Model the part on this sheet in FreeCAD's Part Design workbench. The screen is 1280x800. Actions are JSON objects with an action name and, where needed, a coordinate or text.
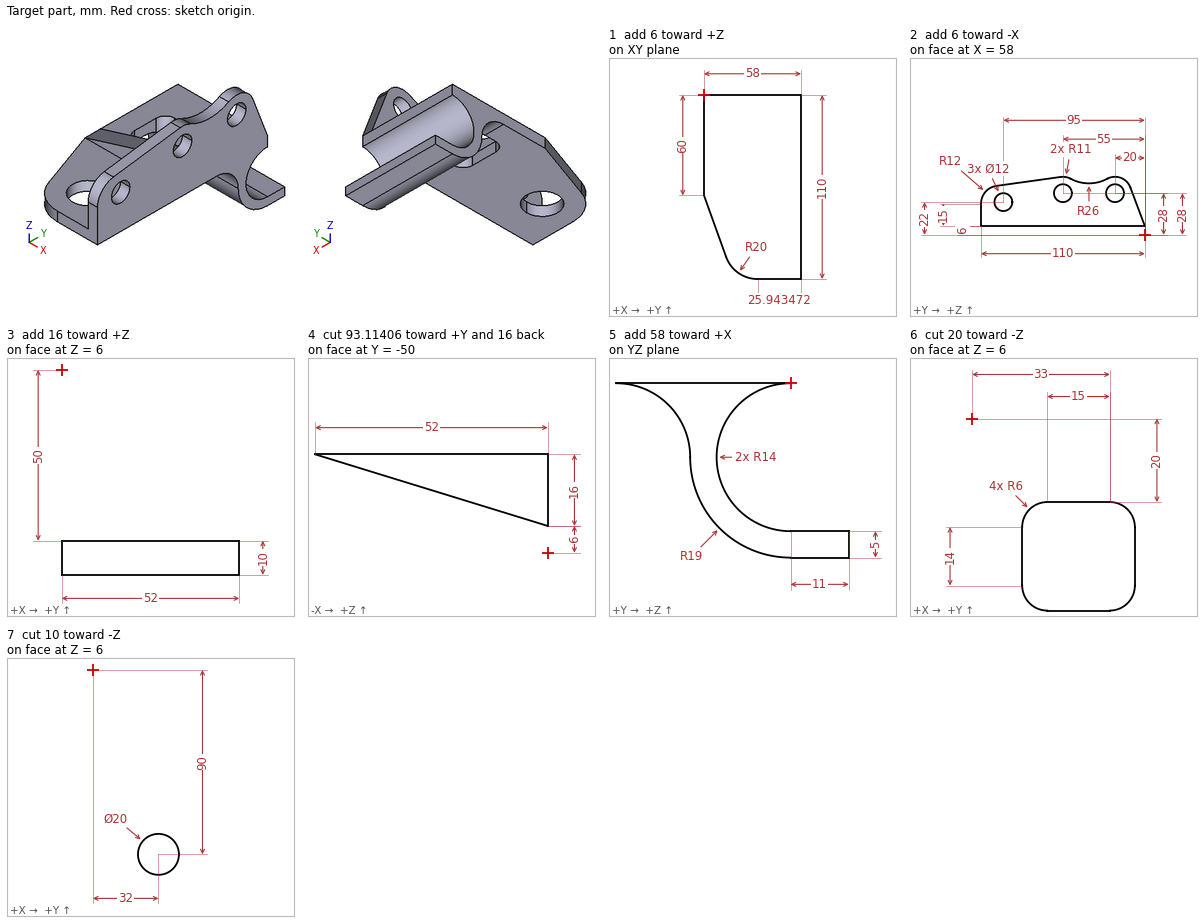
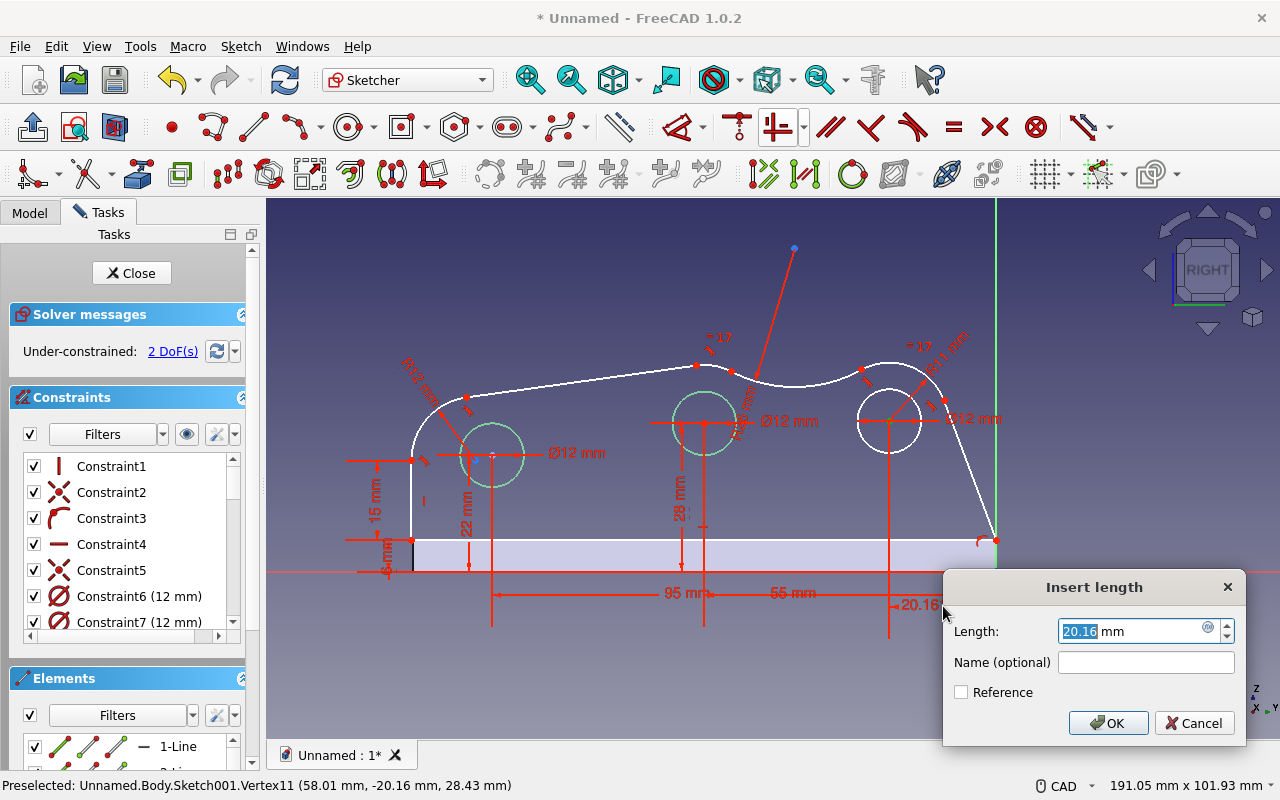
{"action": "type", "text": "20"}
{"action": "key", "text": "Return"}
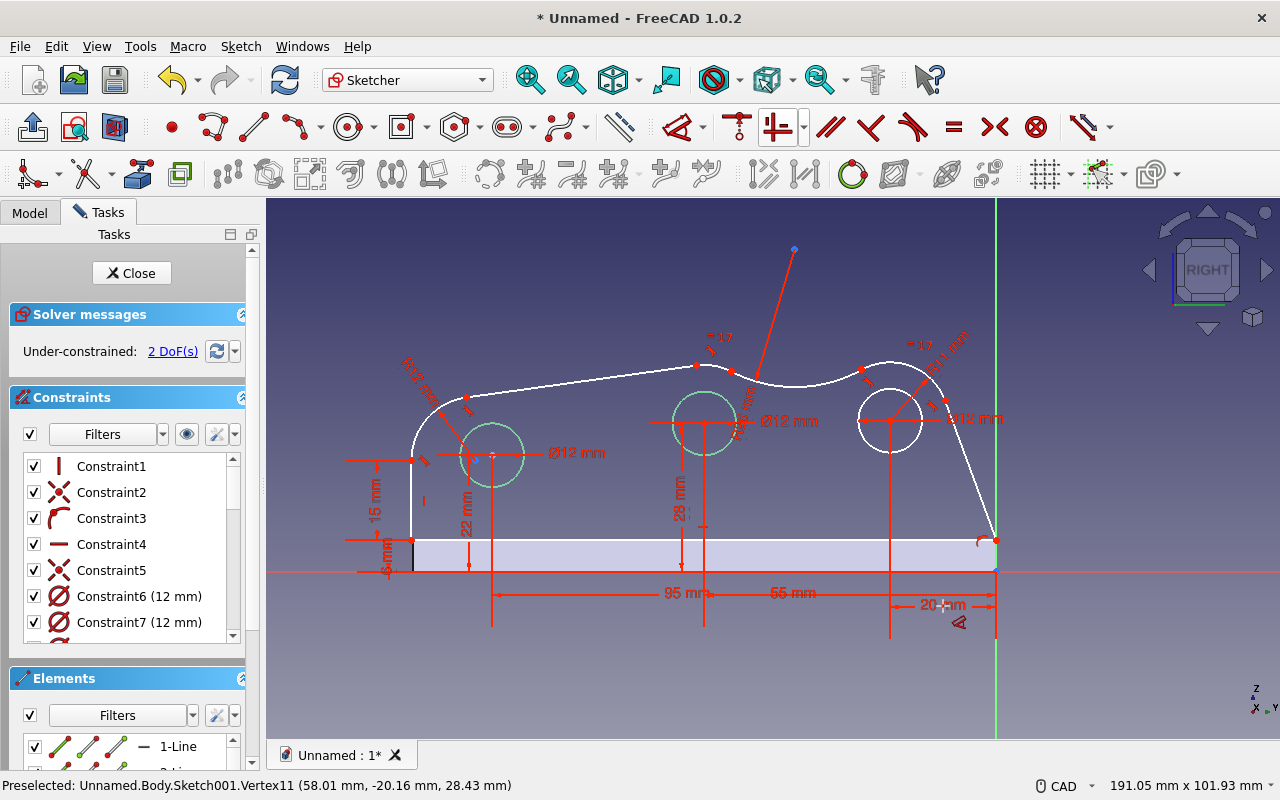
{"action": "left_click", "coordinate": [890, 421]}
{"action": "left_click", "coordinate": [1030, 496]}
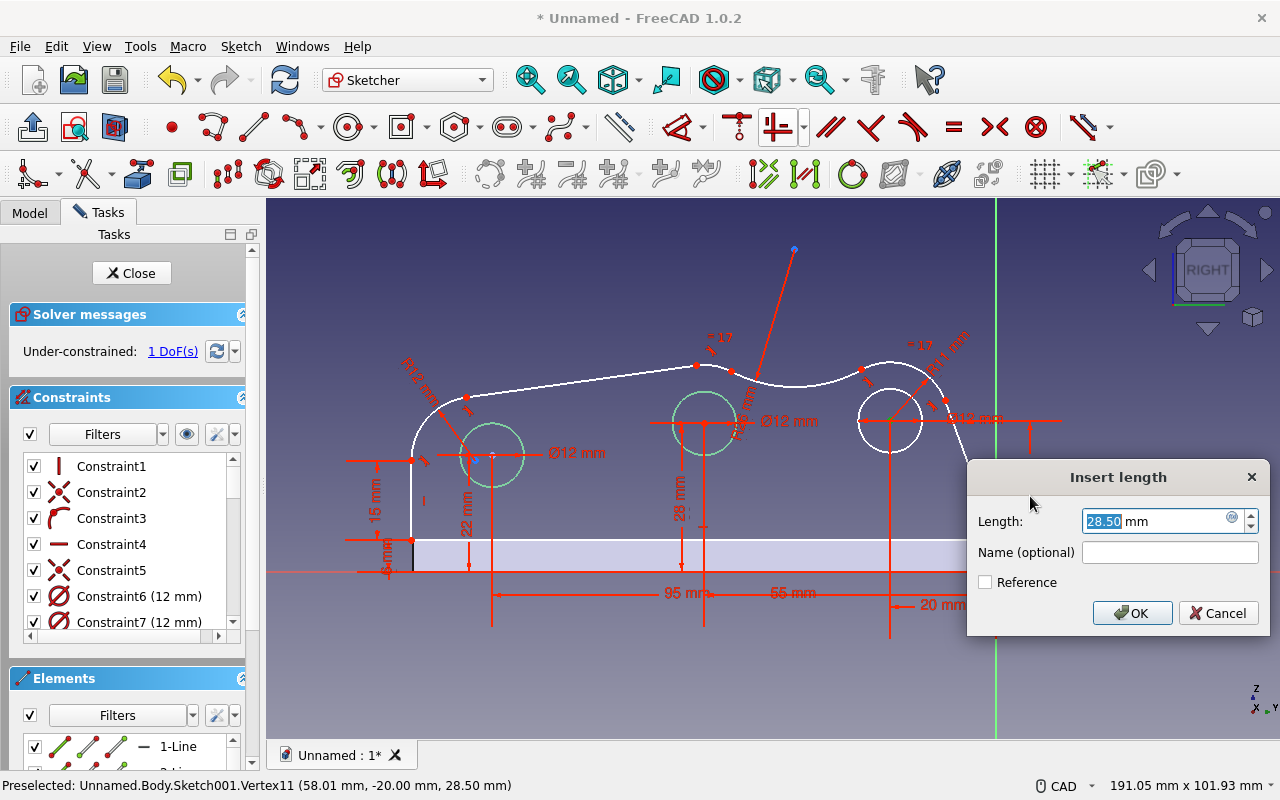
{"action": "type", "text": "28"}
{"action": "key", "text": "Return"}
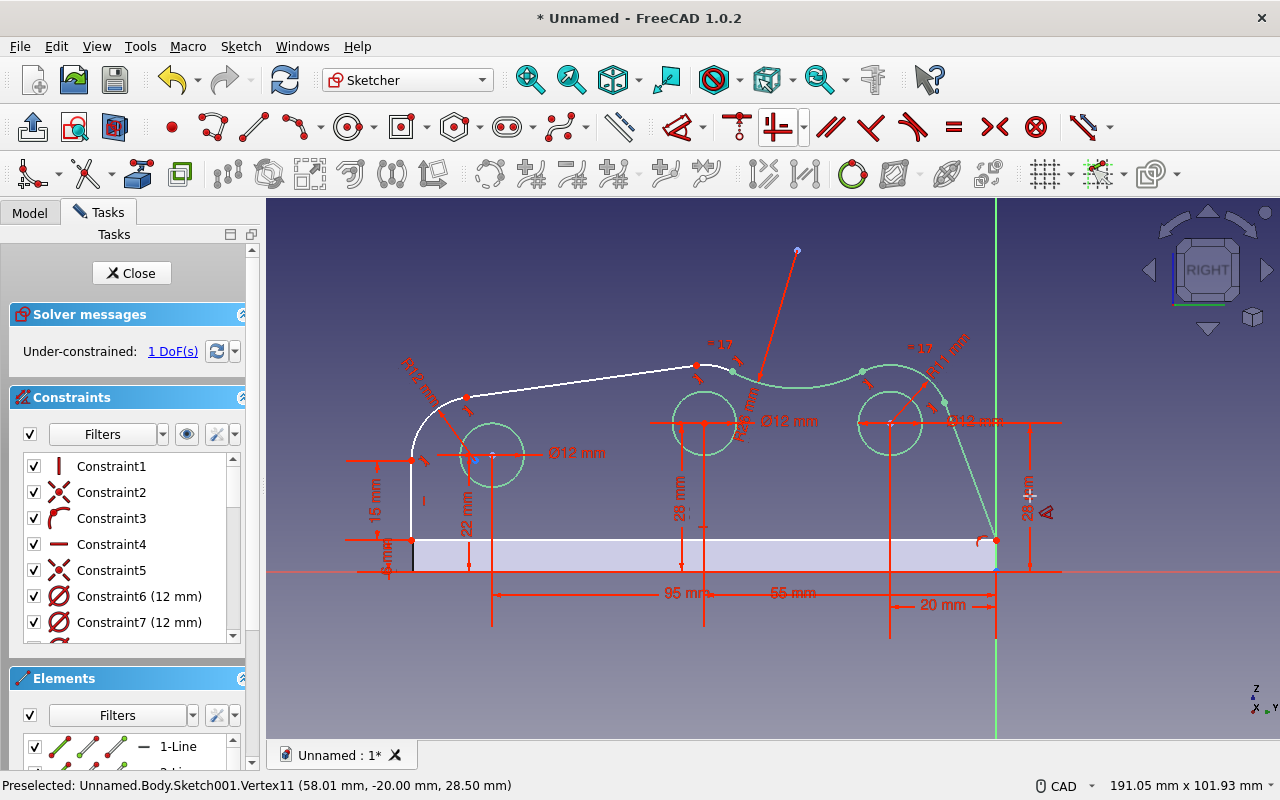
{"action": "left_click", "coordinate": [587, 540]}
{"action": "left_click", "coordinate": [569, 506]}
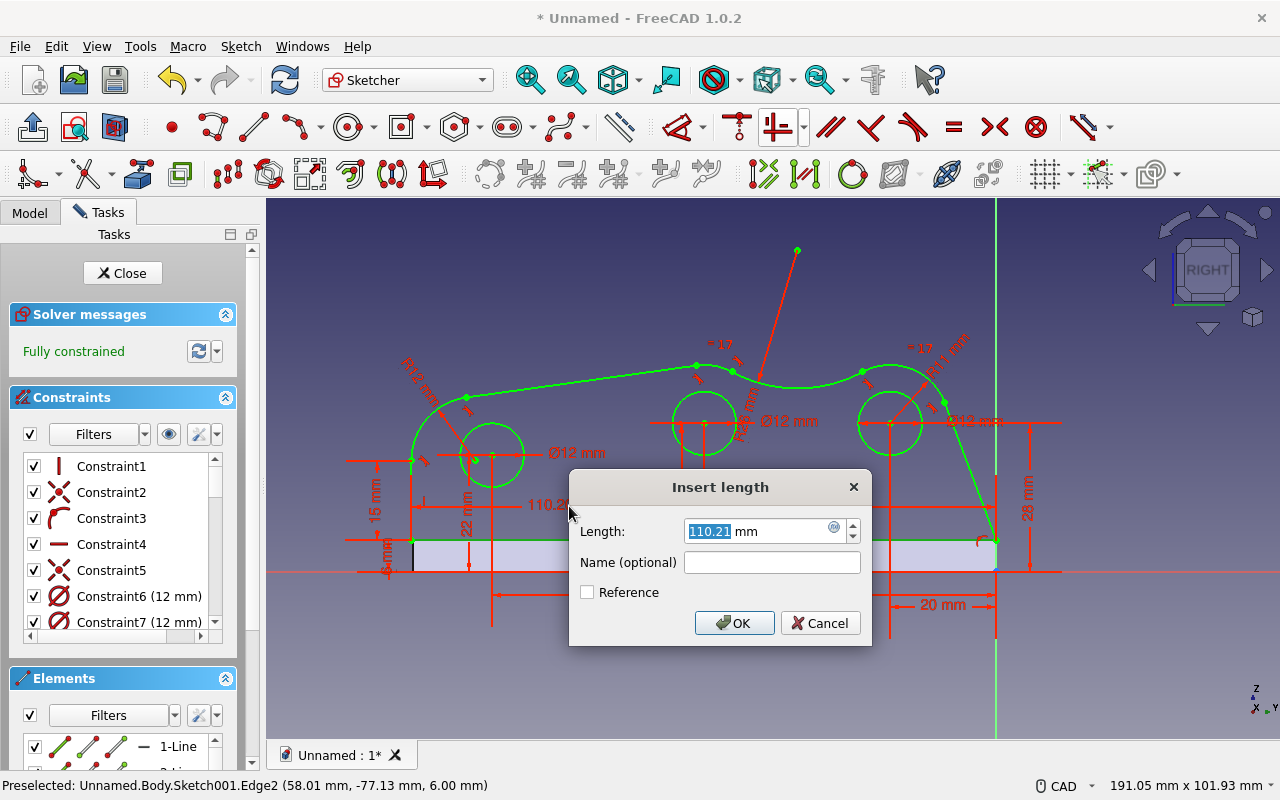
{"action": "type", "text": "110"}
{"action": "key", "text": "Return"}
{"action": "key", "text": "Escape"}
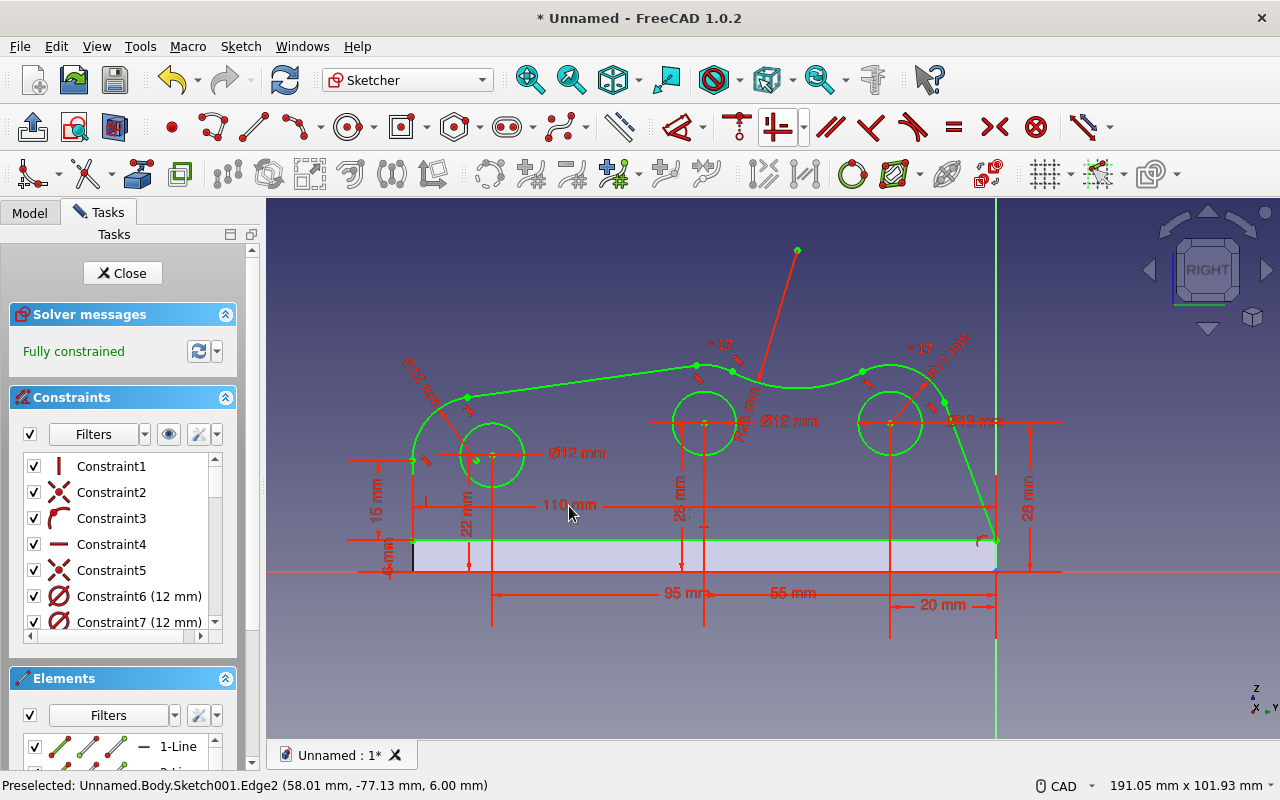
{"action": "left_click", "coordinate": [123, 273]}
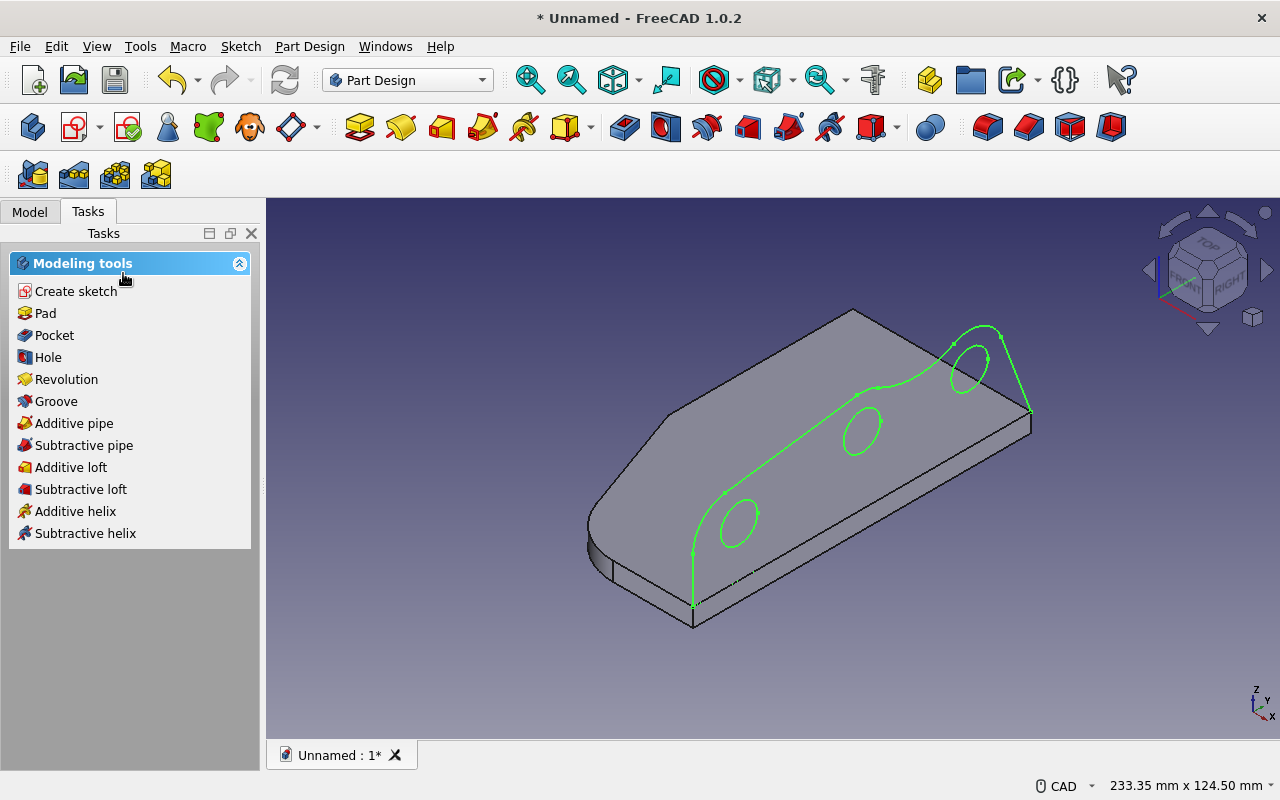
{"action": "left_click", "coordinate": [360, 128]}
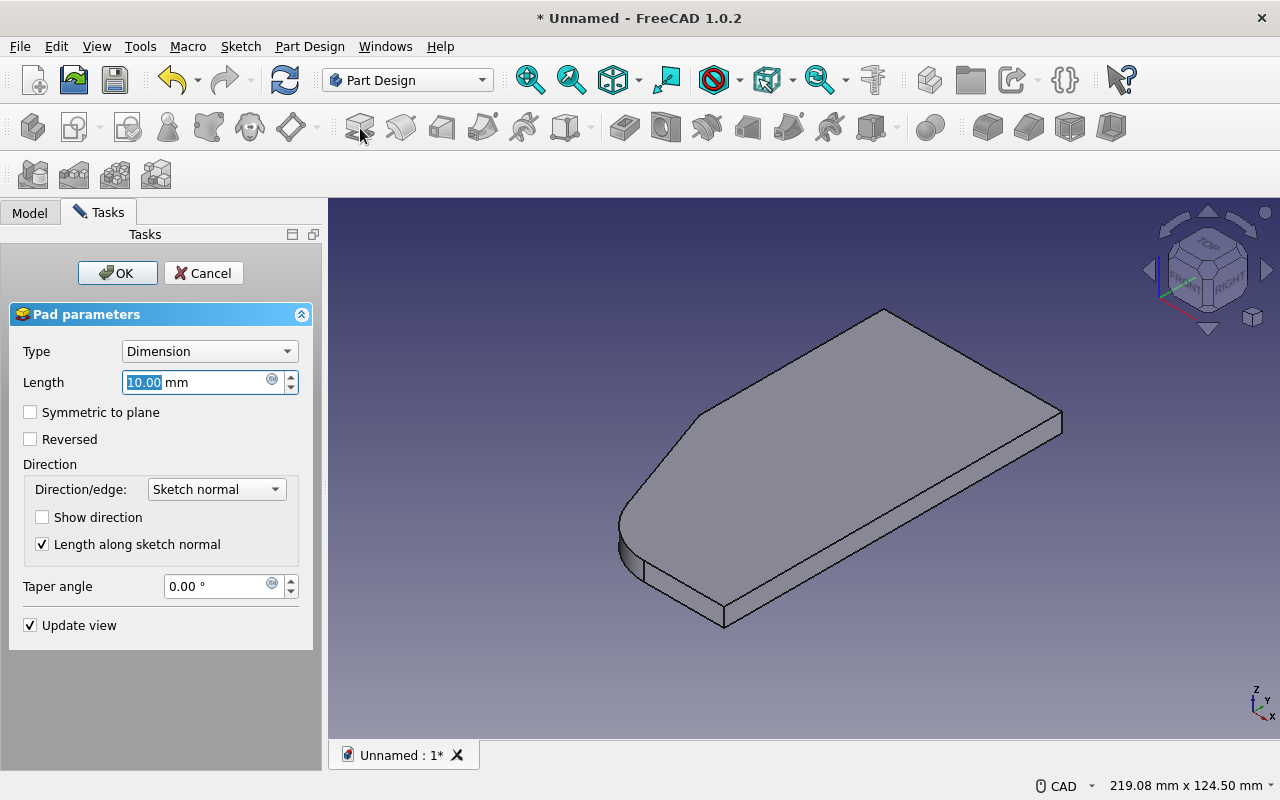
{"action": "type", "text": "6"}
{"action": "key", "text": "Tab"}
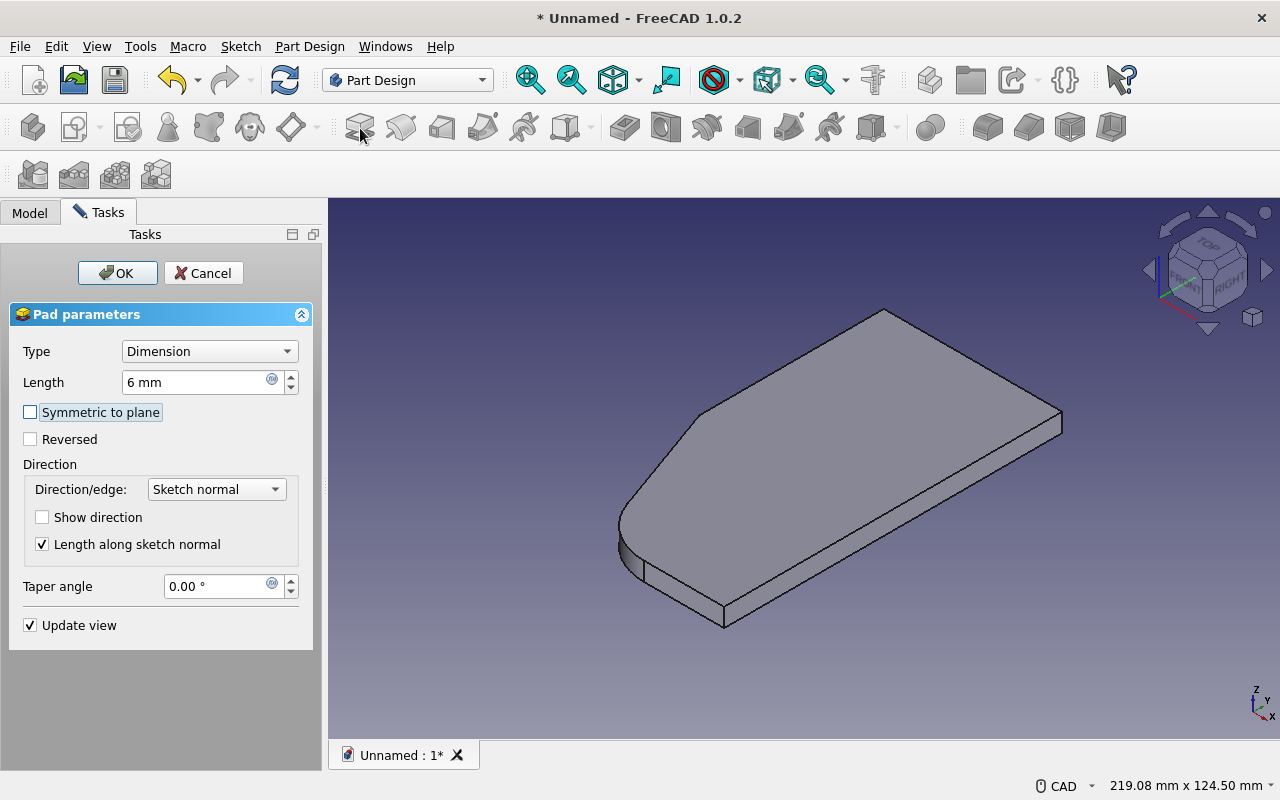
{"action": "left_click", "coordinate": [31, 439]}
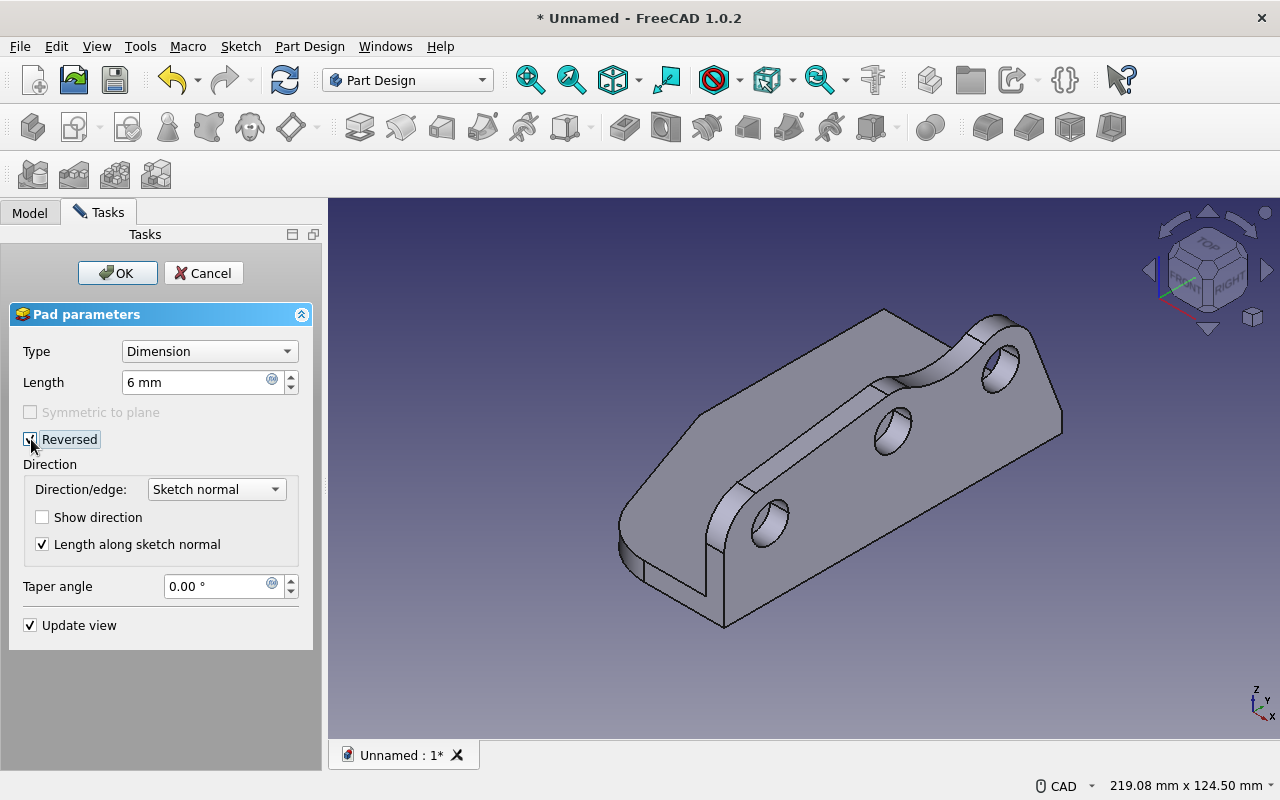
{"action": "left_click", "coordinate": [118, 273]}